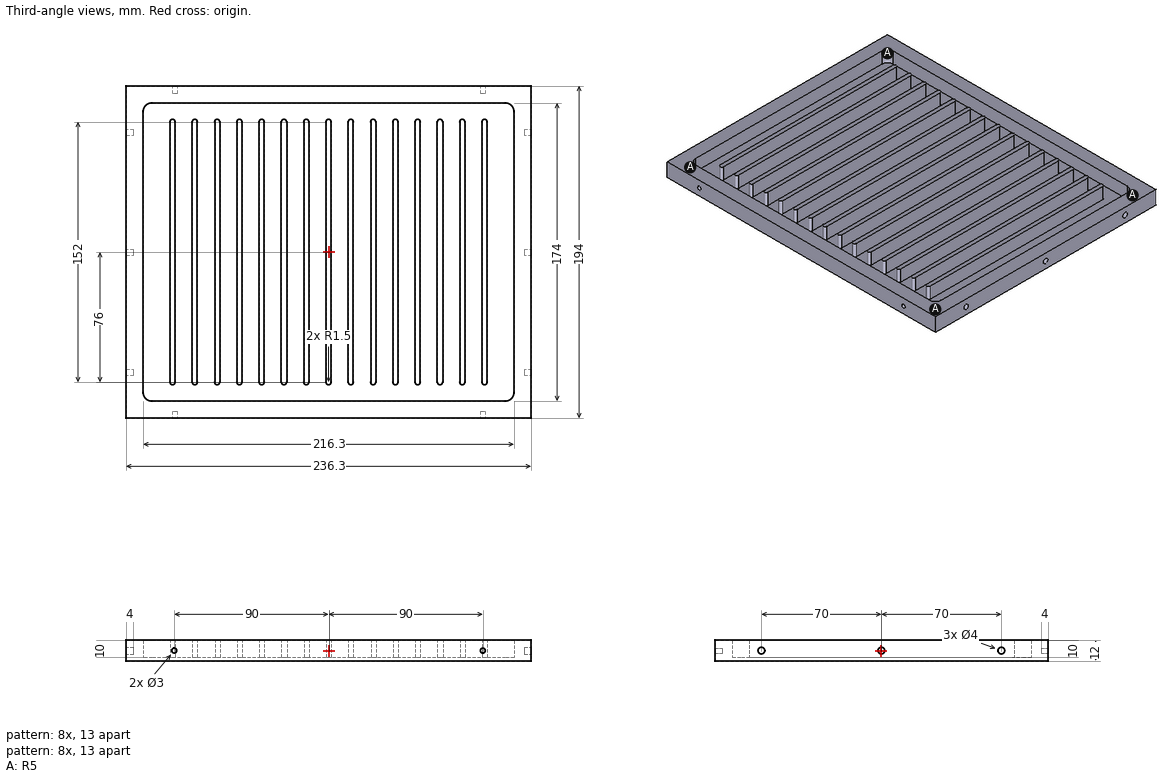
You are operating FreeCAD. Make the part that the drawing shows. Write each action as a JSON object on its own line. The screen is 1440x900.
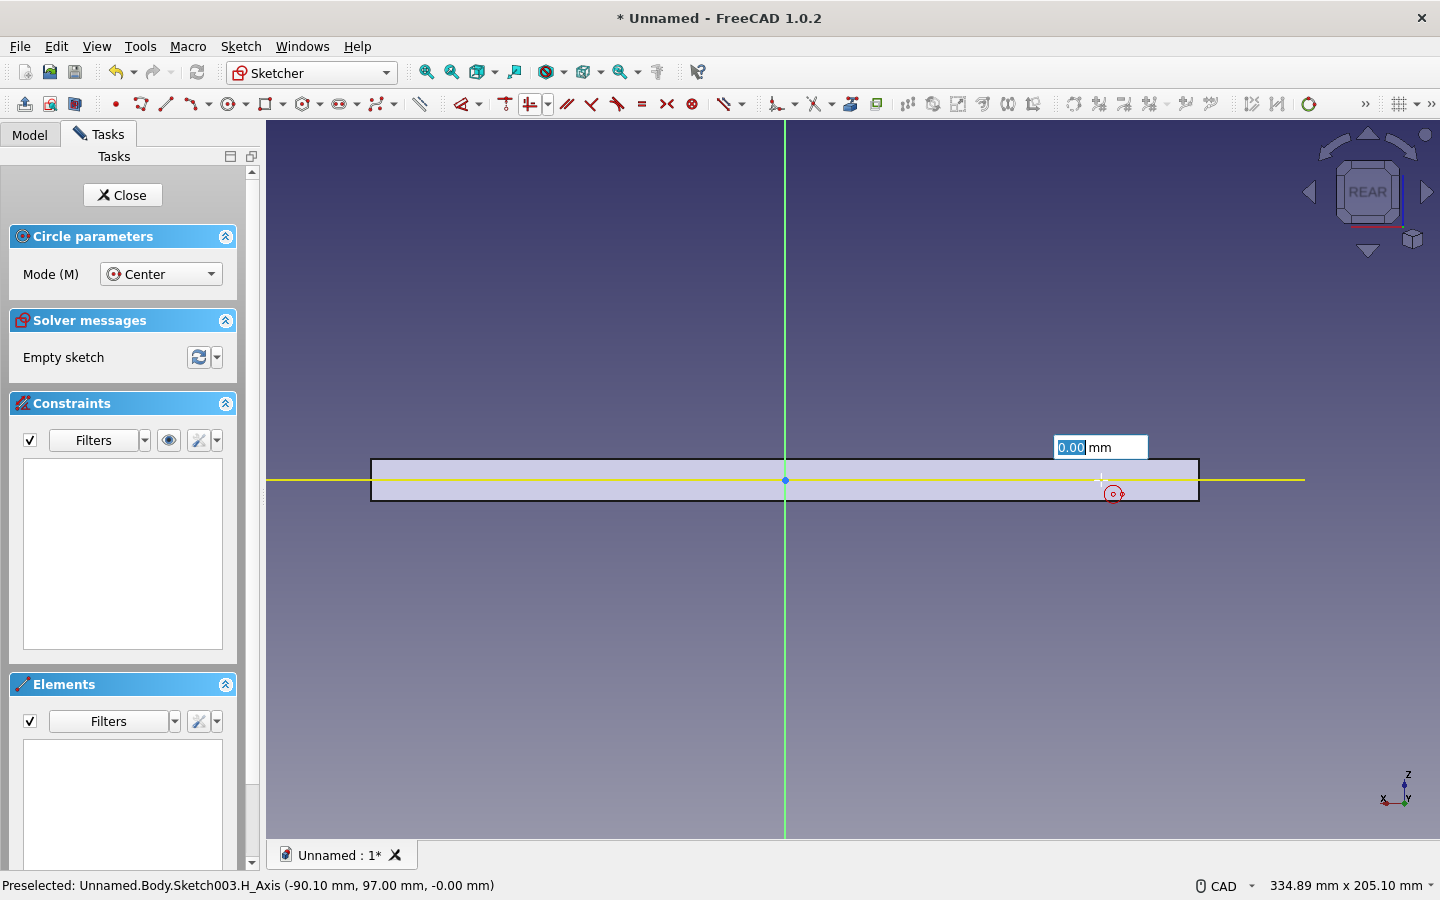
{"action": "scroll", "coordinate": [1099, 485], "scroll_direction": "up", "scroll_amount": 6}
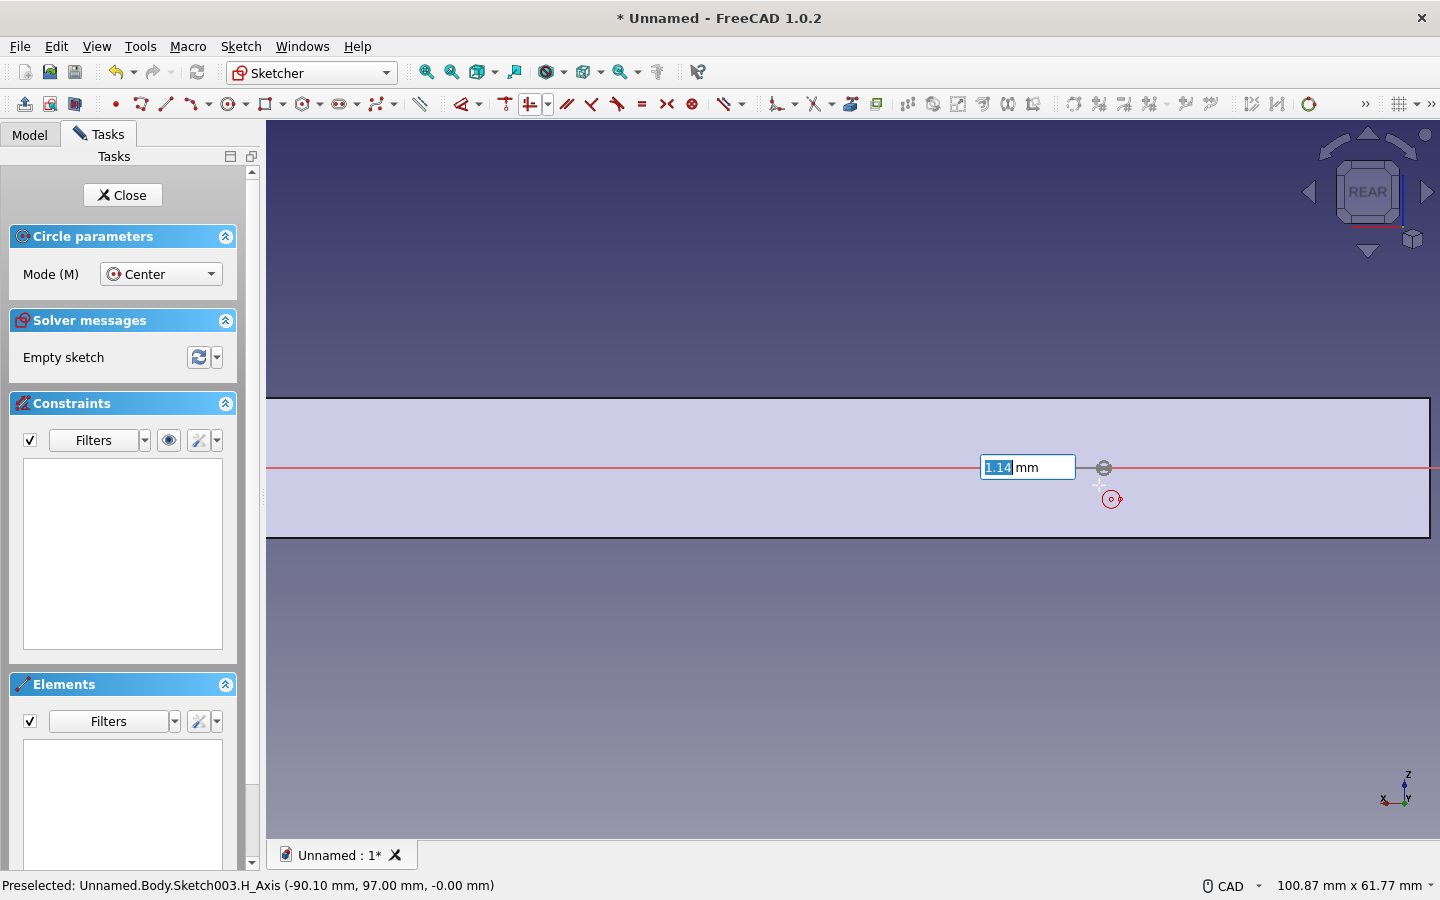
{"action": "left_click", "coordinate": [1097, 485]}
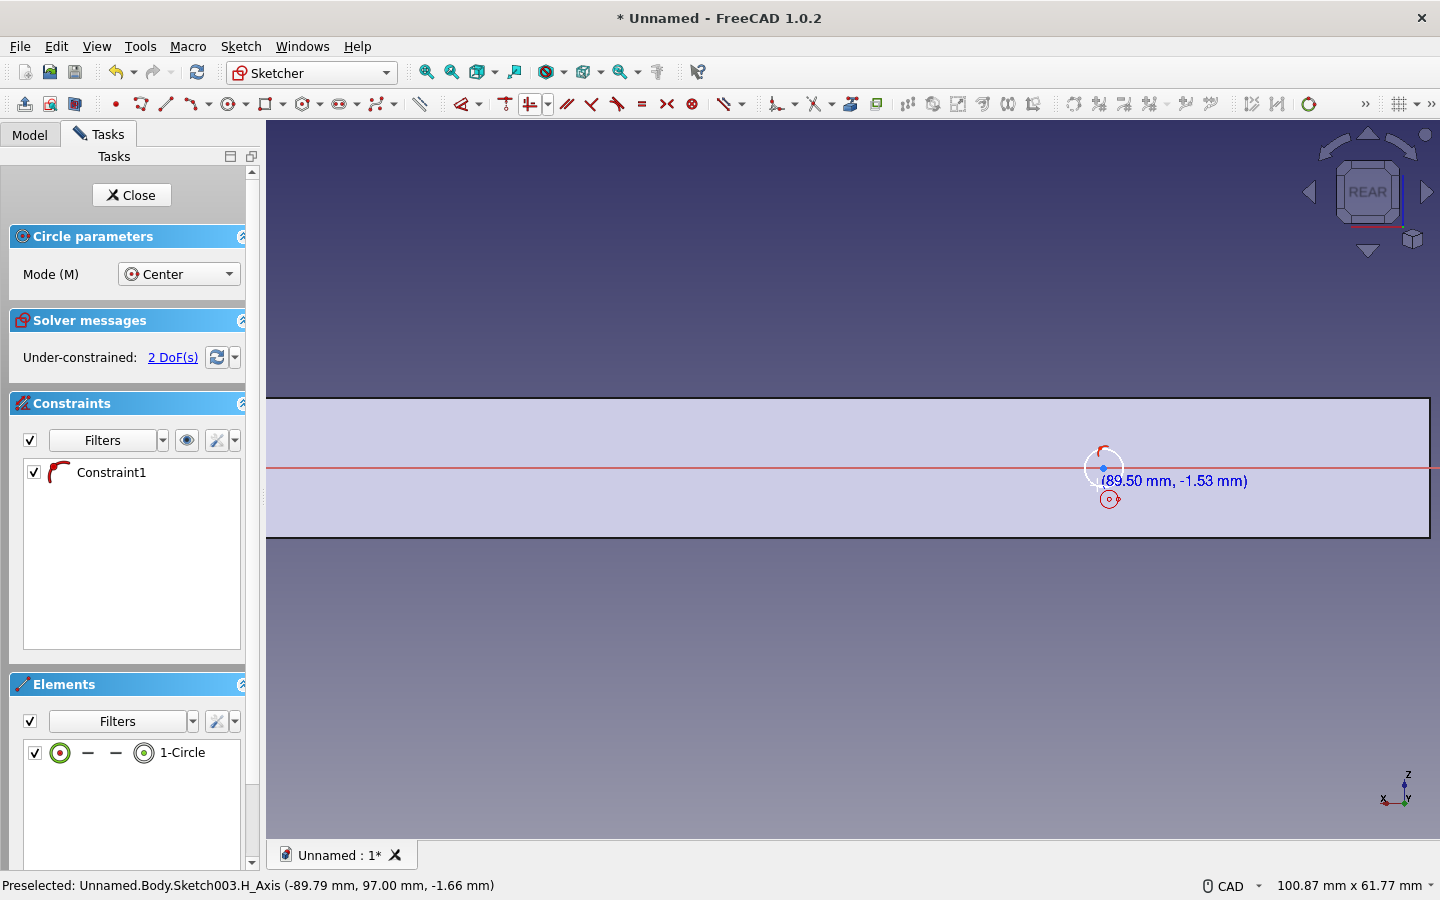
{"action": "scroll", "coordinate": [1099, 484], "scroll_direction": "down", "scroll_amount": 6}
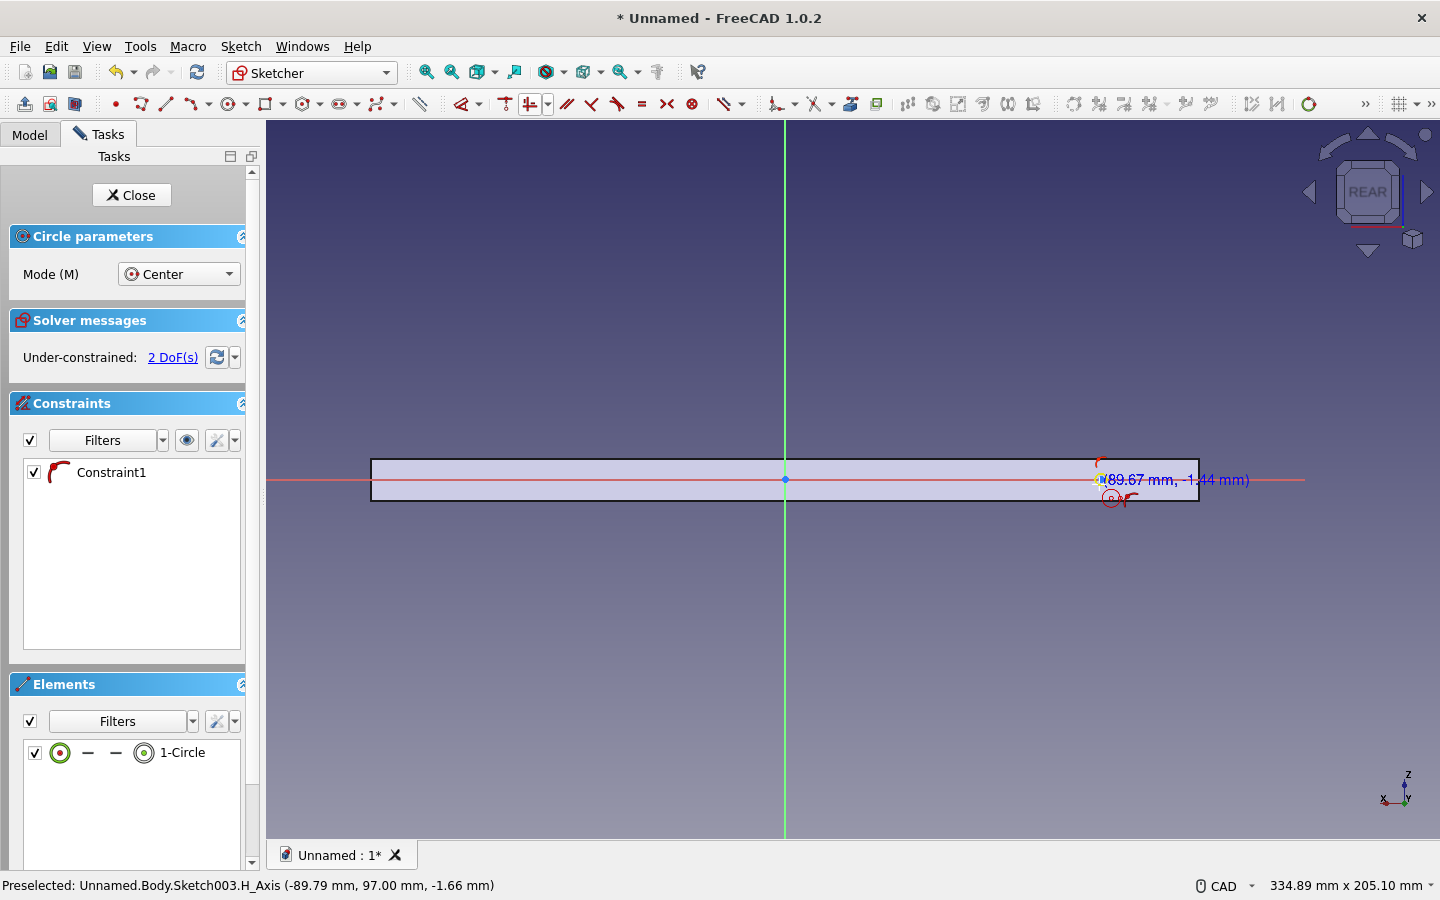
{"action": "scroll", "coordinate": [470, 480], "scroll_direction": "up", "scroll_amount": 8}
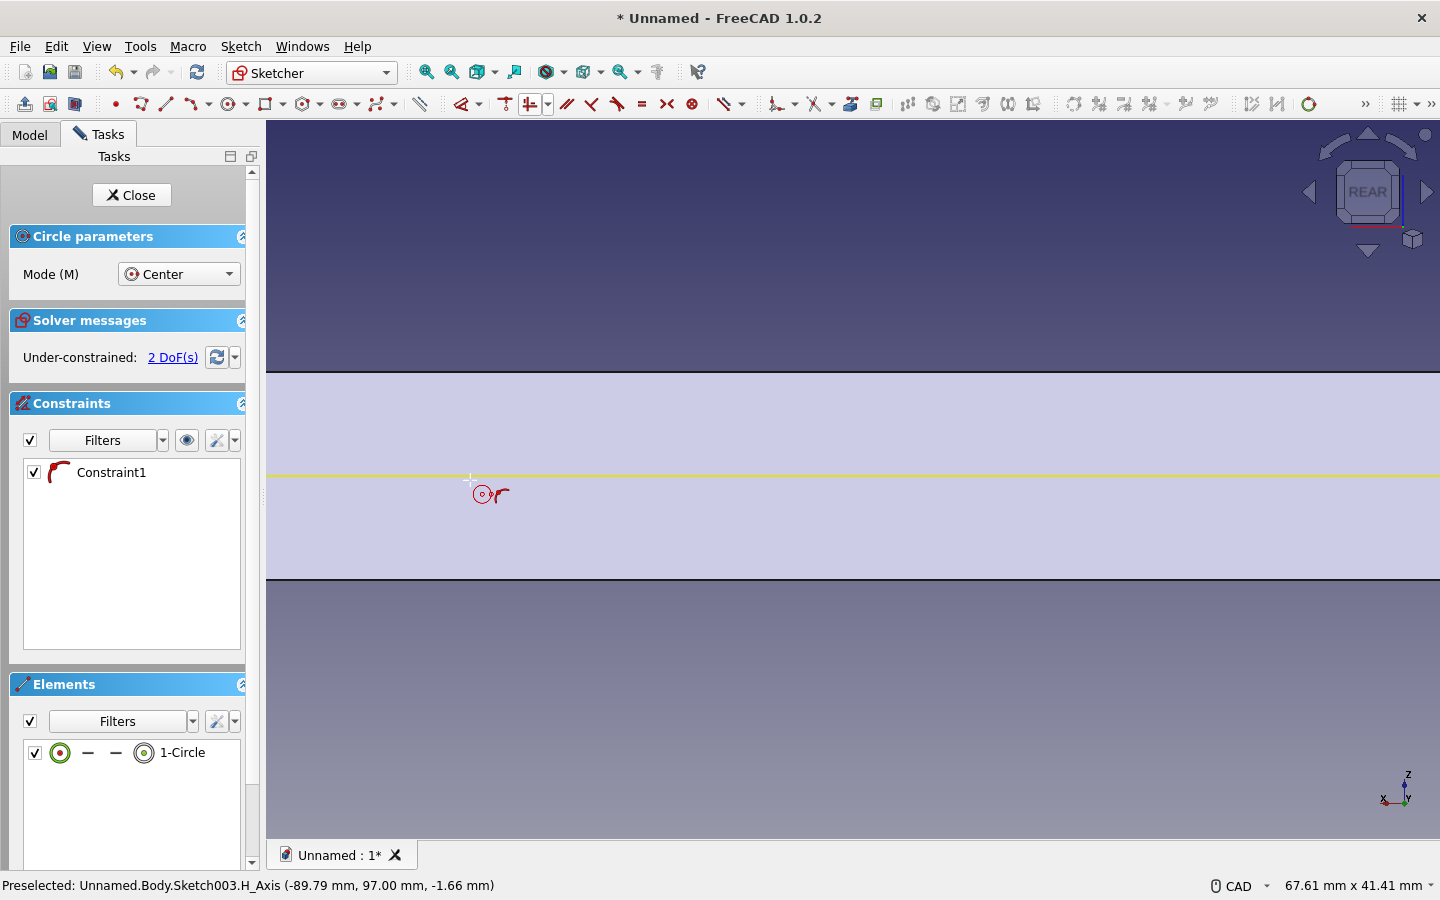
{"action": "scroll", "coordinate": [469, 480], "scroll_direction": "down", "scroll_amount": 8}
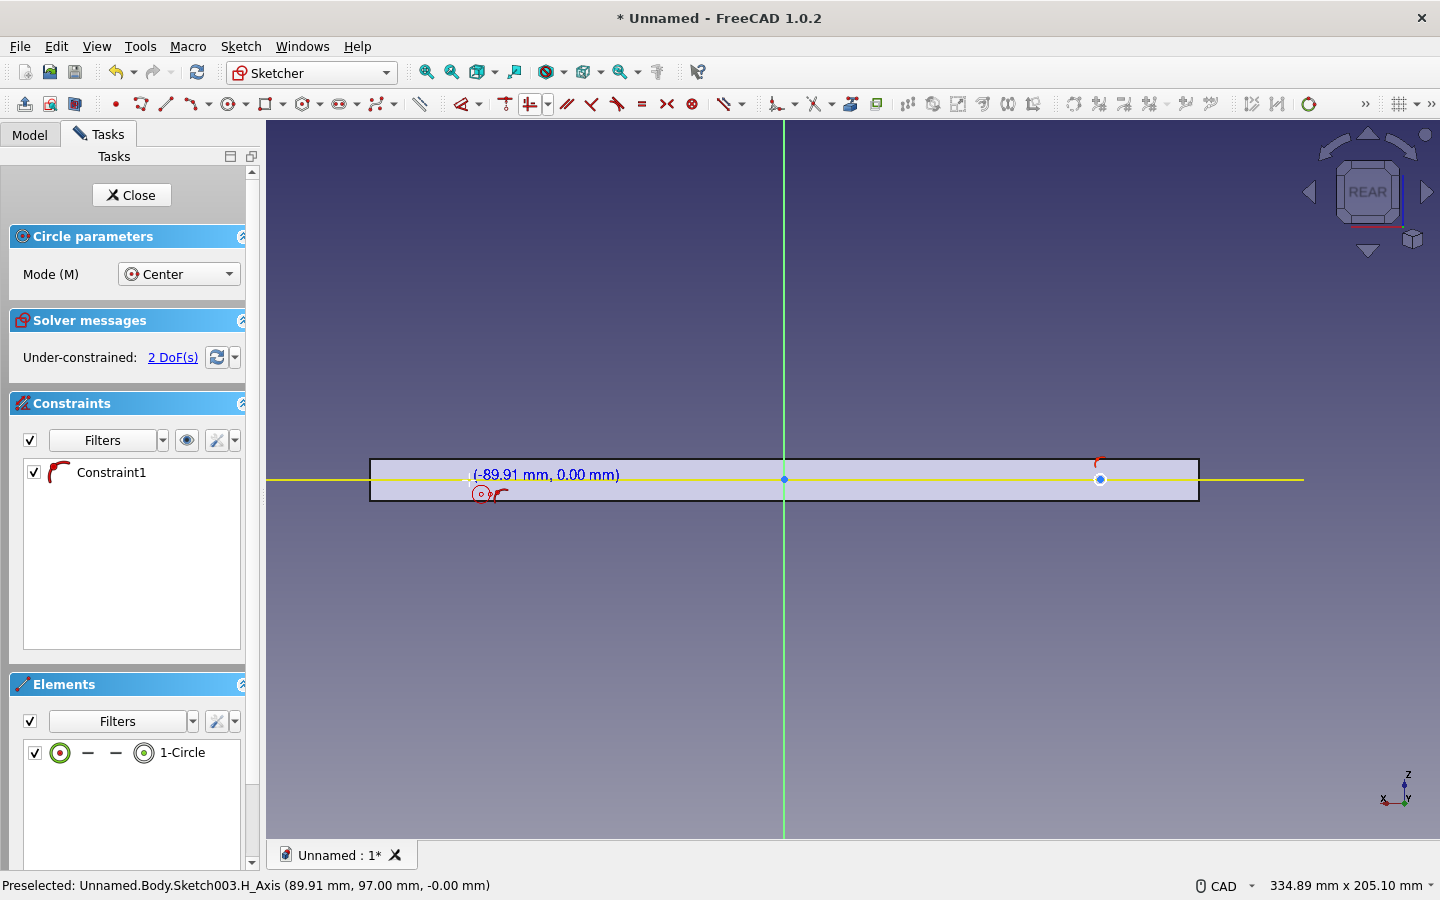
{"action": "left_click", "coordinate": [469, 480]}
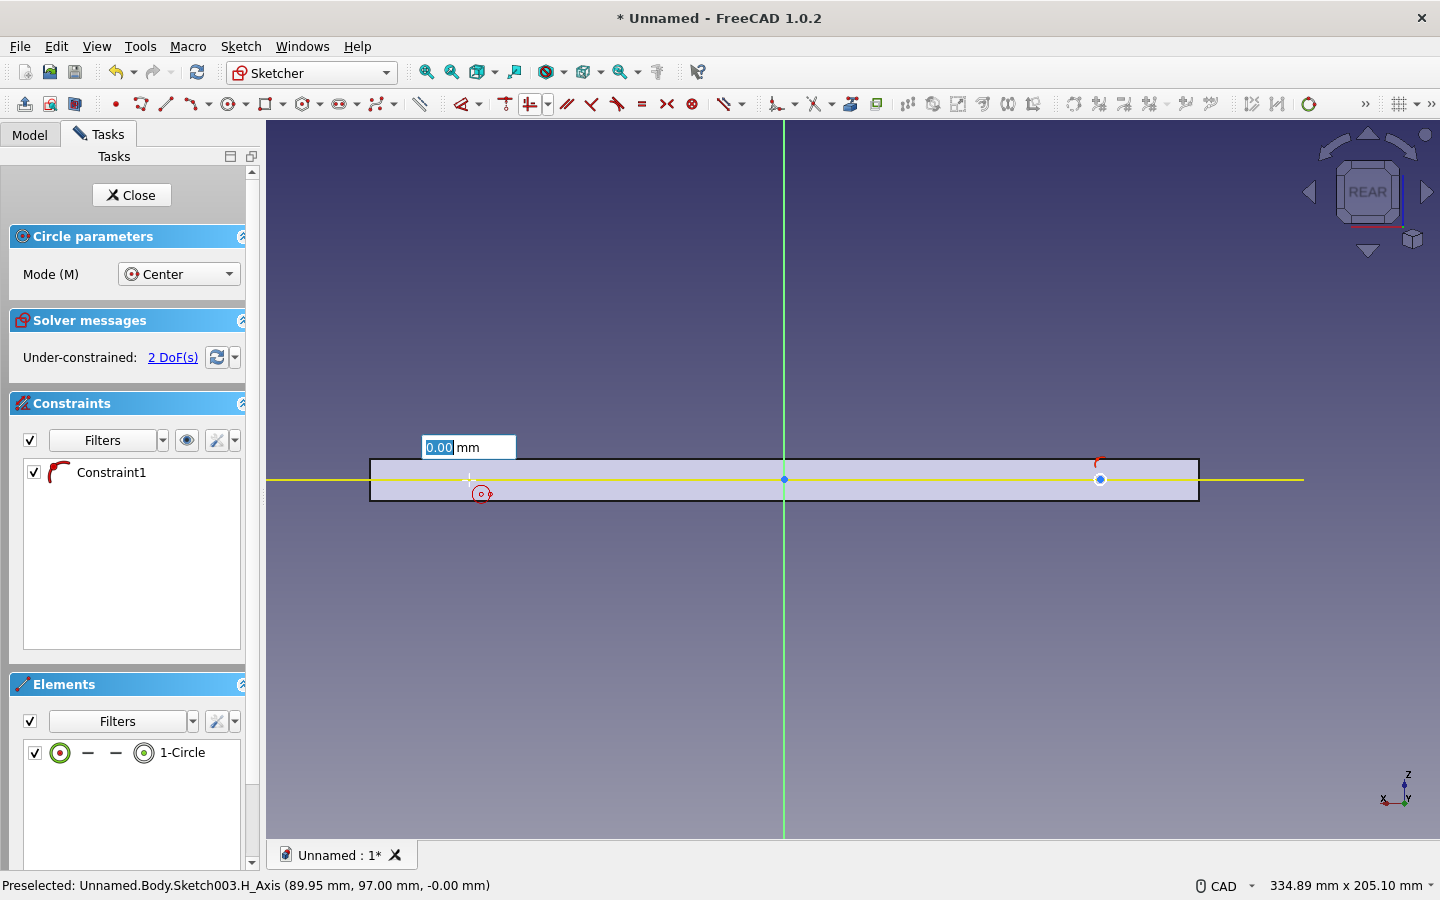
{"action": "scroll", "coordinate": [467, 485], "scroll_direction": "up", "scroll_amount": 6}